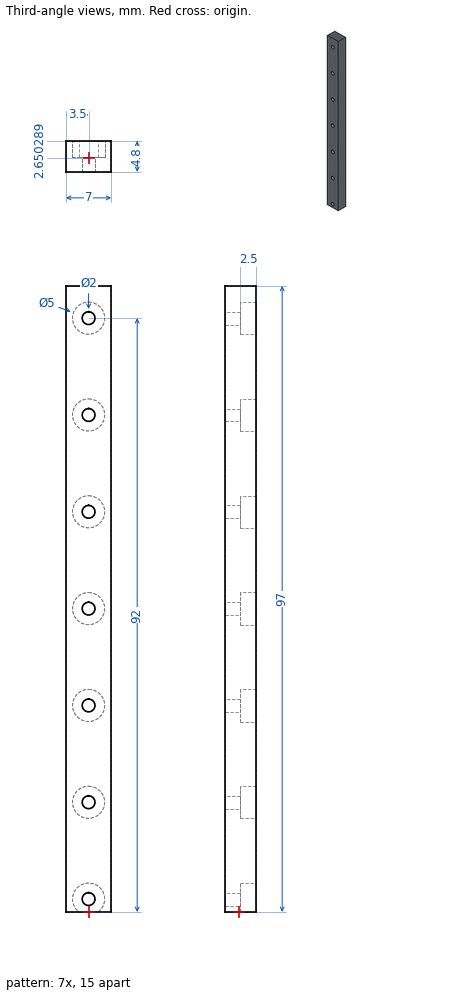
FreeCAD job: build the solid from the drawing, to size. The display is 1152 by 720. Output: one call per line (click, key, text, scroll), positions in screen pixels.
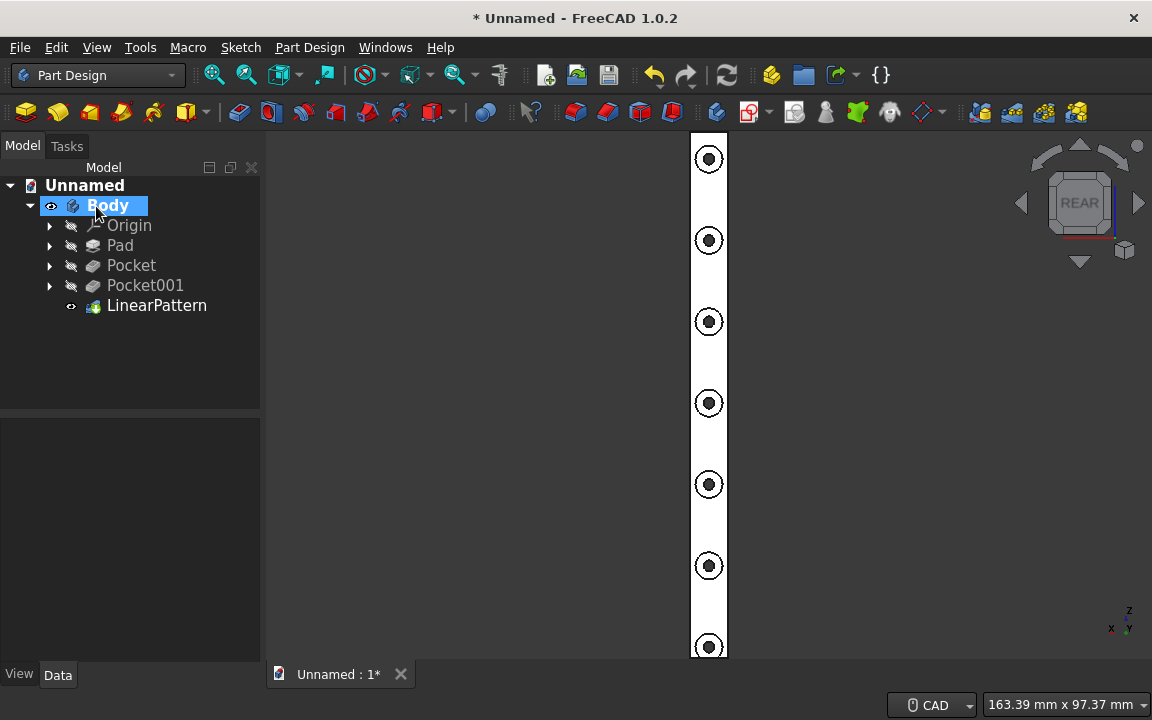
key(0)